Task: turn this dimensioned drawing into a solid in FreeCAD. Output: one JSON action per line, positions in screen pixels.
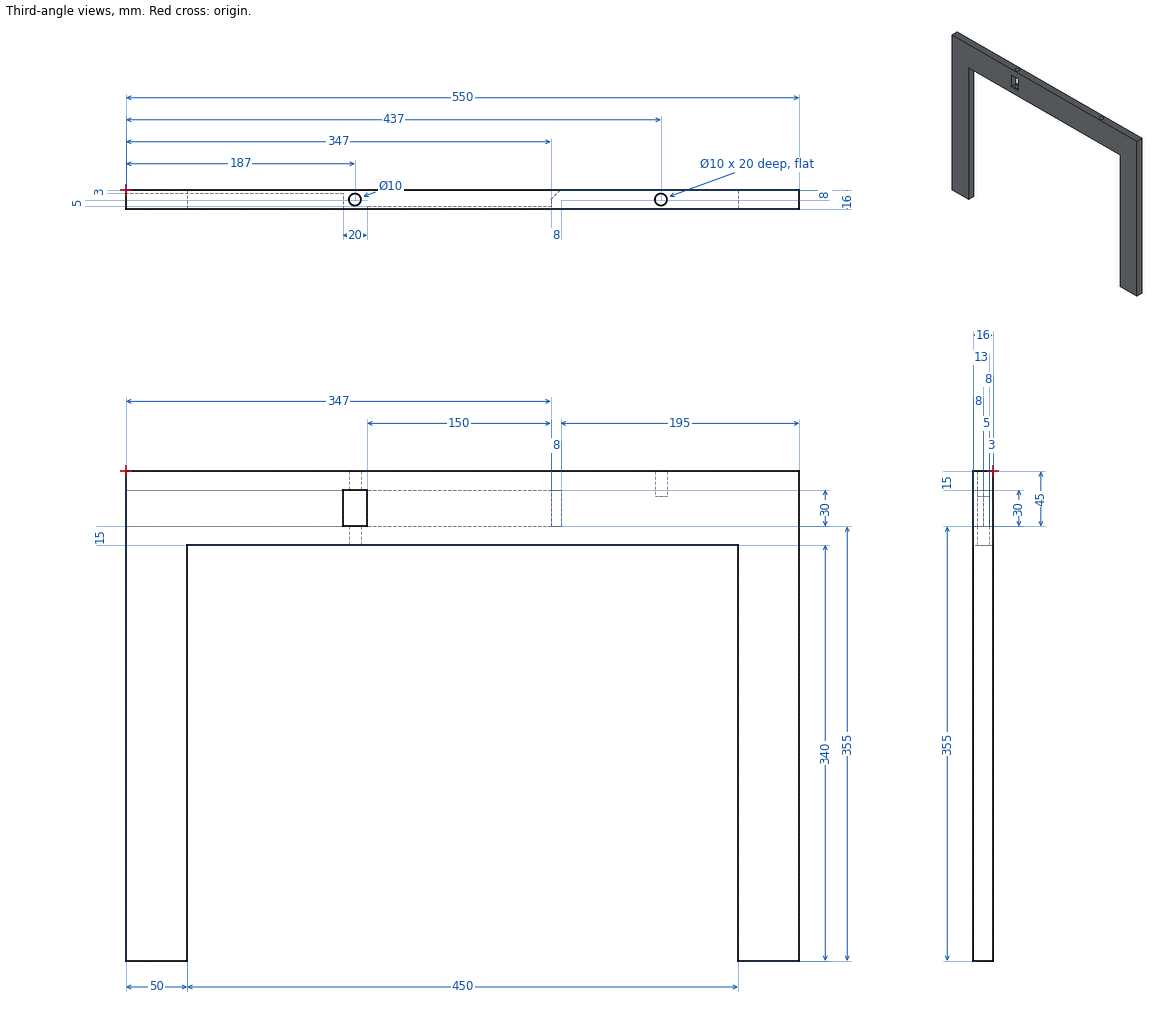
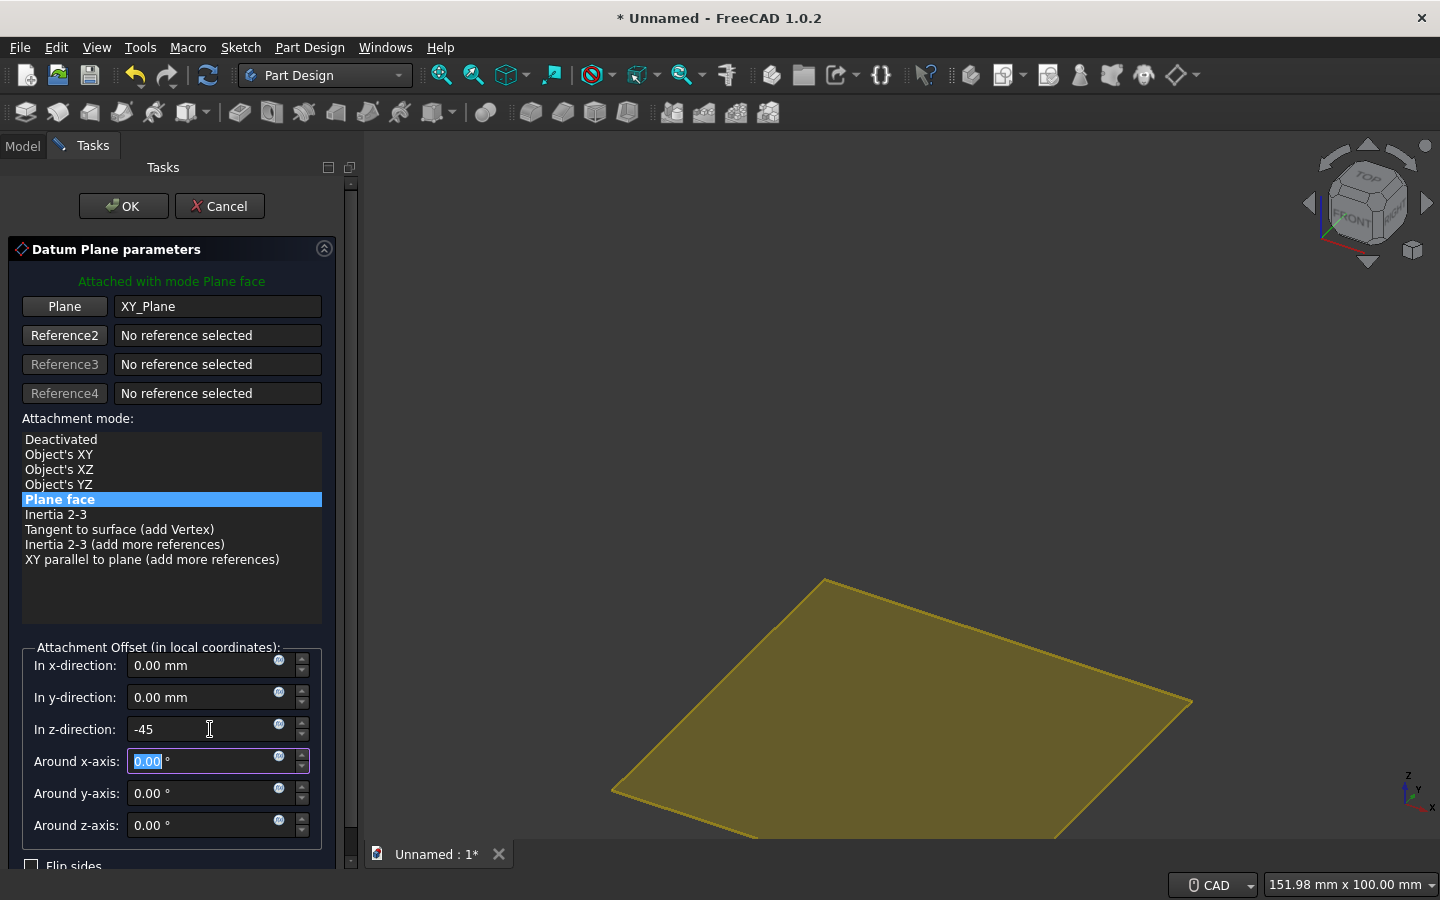
{"action": "left_click", "coordinate": [124, 206]}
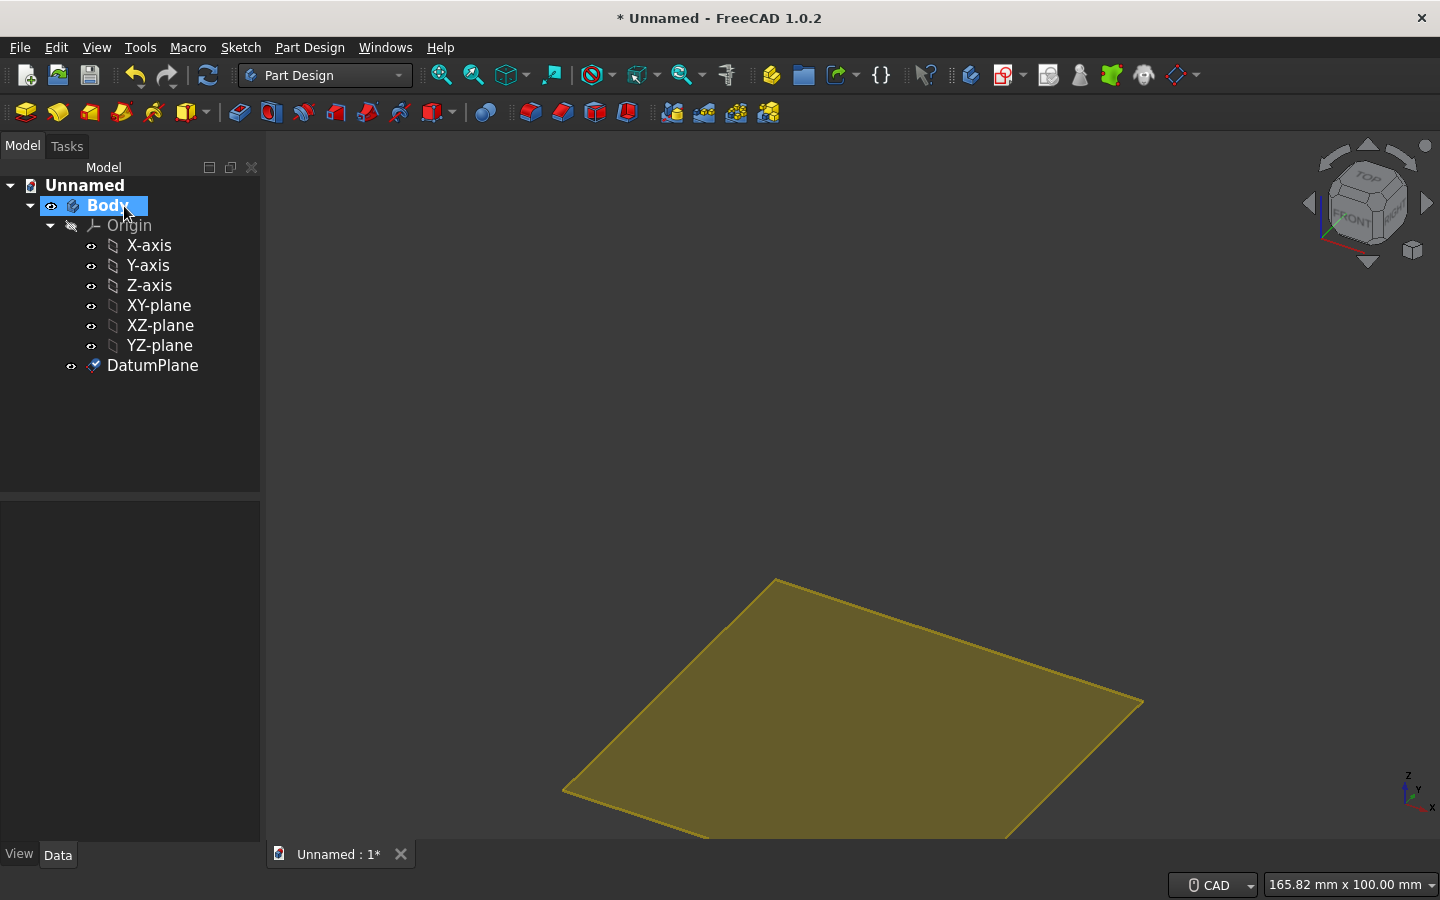
{"action": "left_click", "coordinate": [116, 366]}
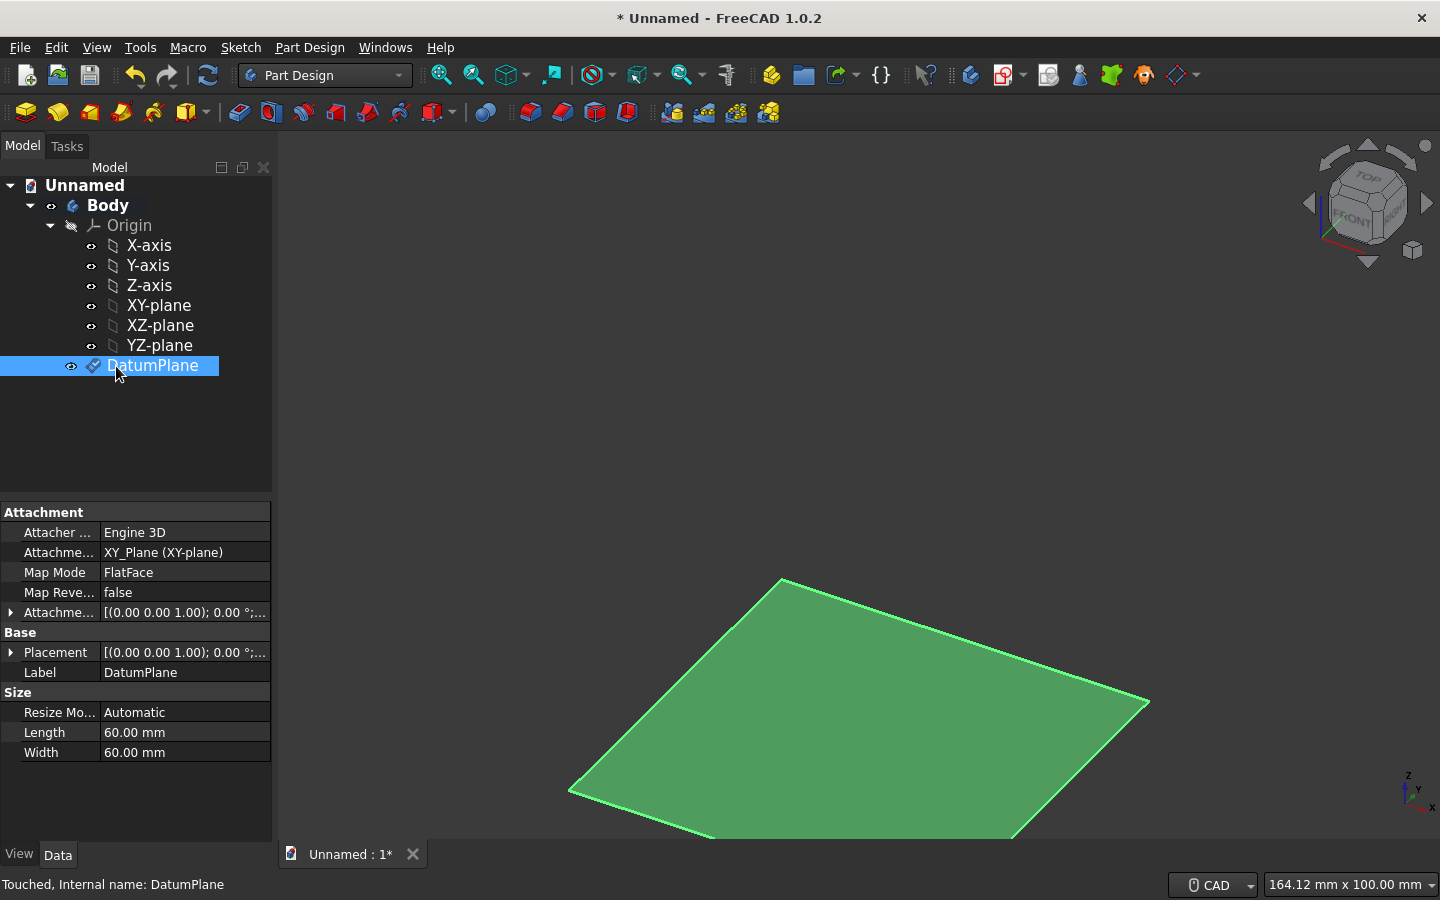
{"action": "left_click", "coordinate": [1004, 76]}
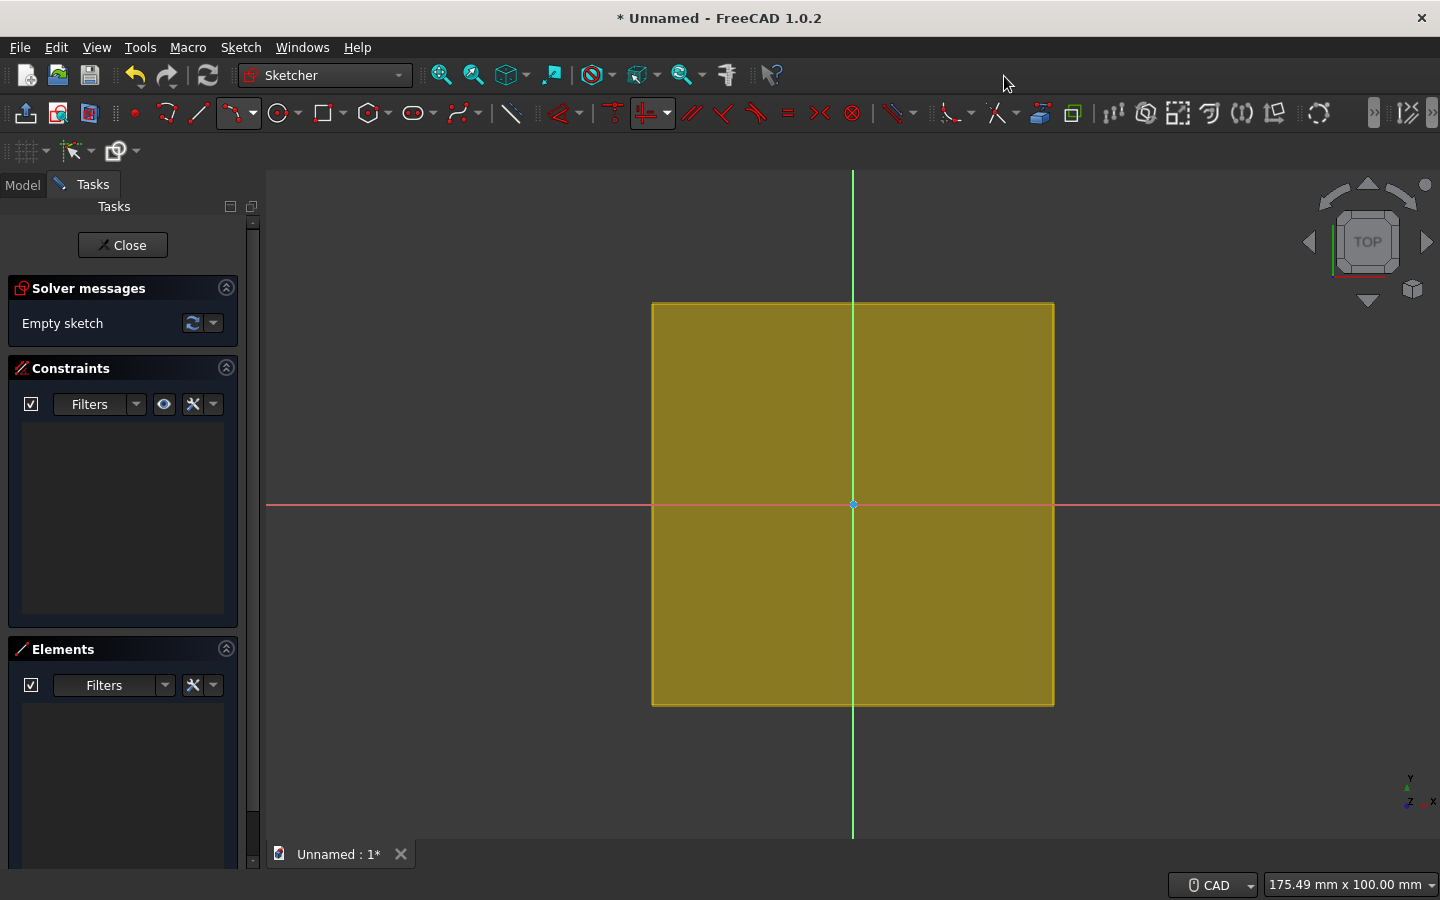
{"action": "scroll", "coordinate": [784, 504], "scroll_direction": "down", "scroll_amount": 5}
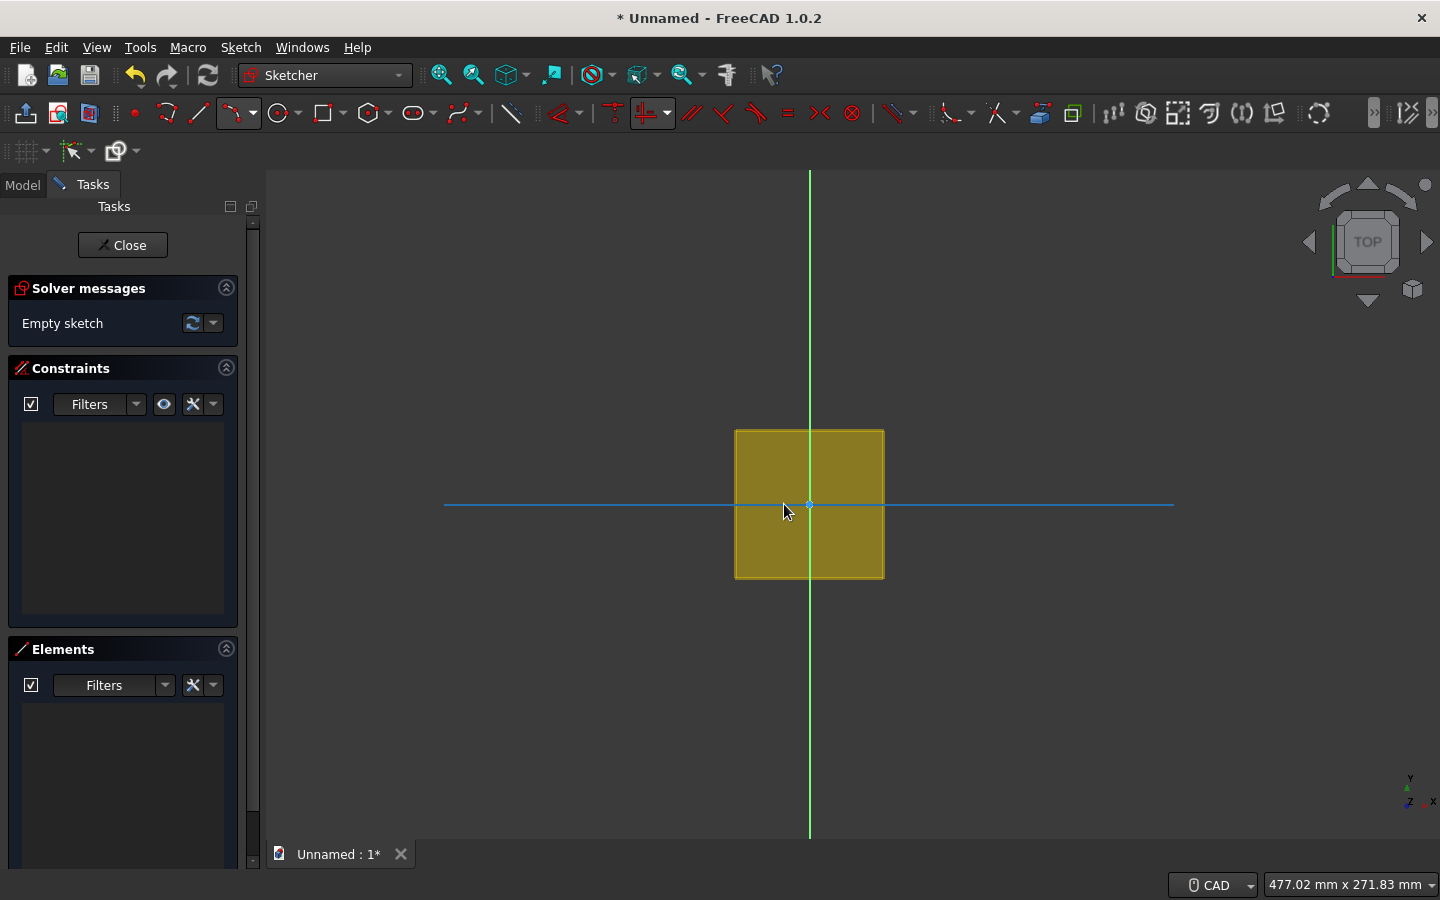
{"action": "scroll", "coordinate": [784, 504], "scroll_direction": "down", "scroll_amount": 5}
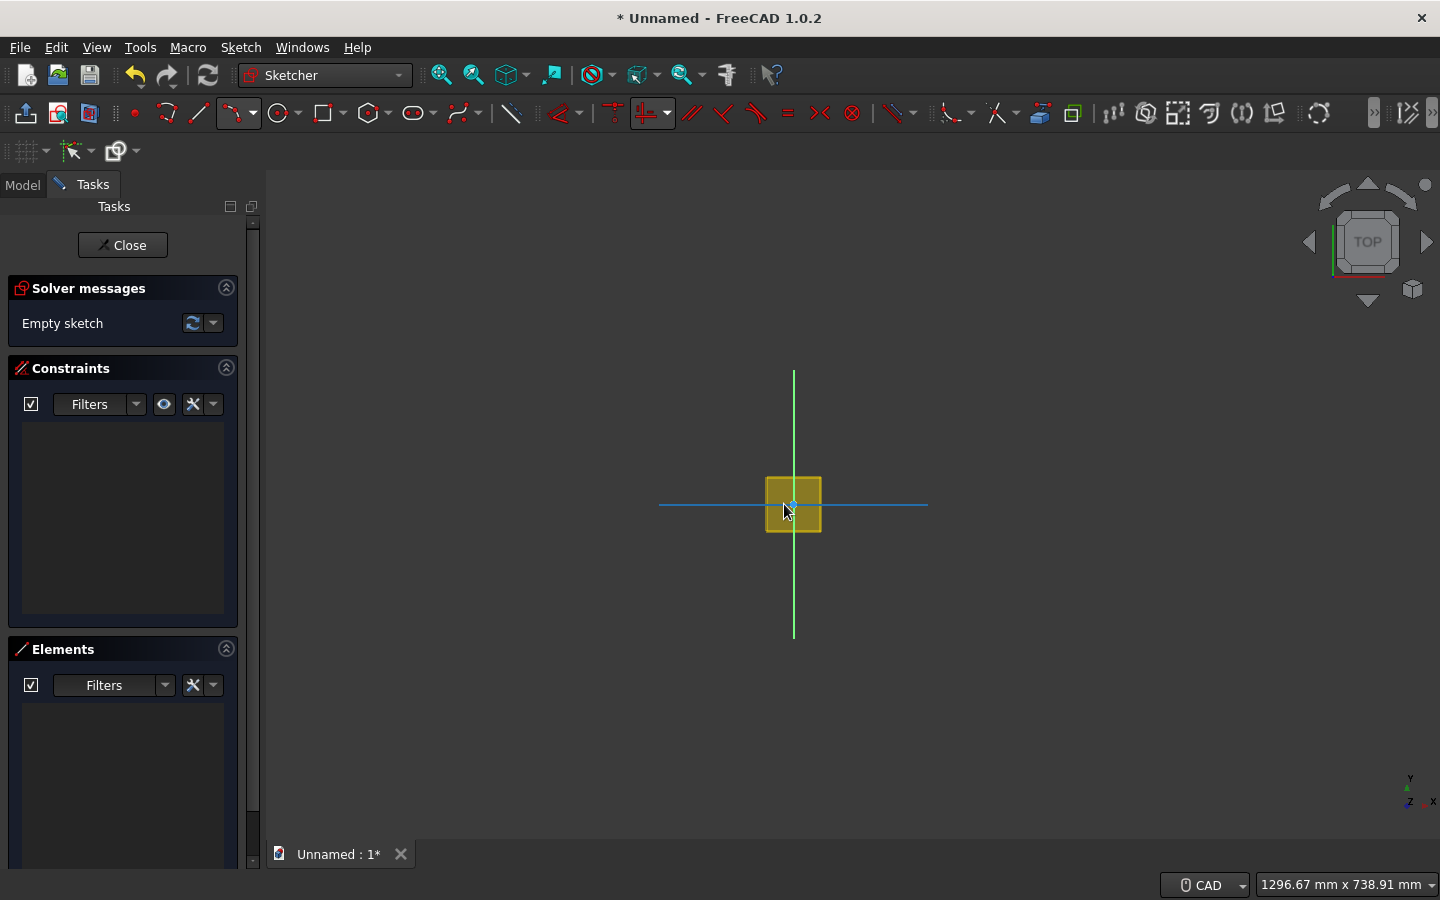
{"action": "scroll", "coordinate": [1129, 508], "scroll_direction": "up", "scroll_amount": 15}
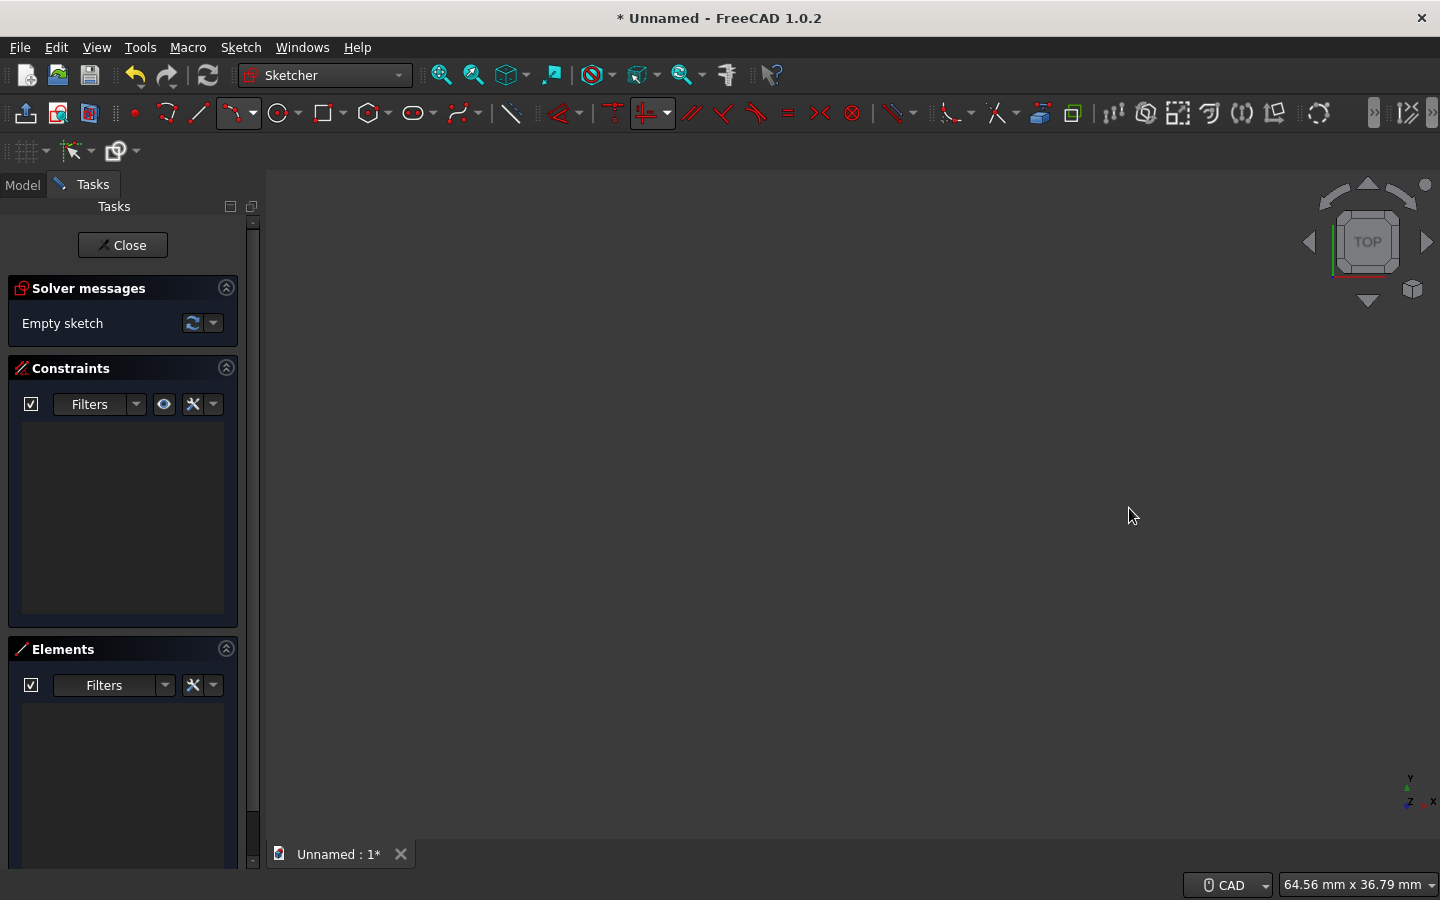
{"action": "scroll", "coordinate": [752, 499], "scroll_direction": "up", "scroll_amount": 5}